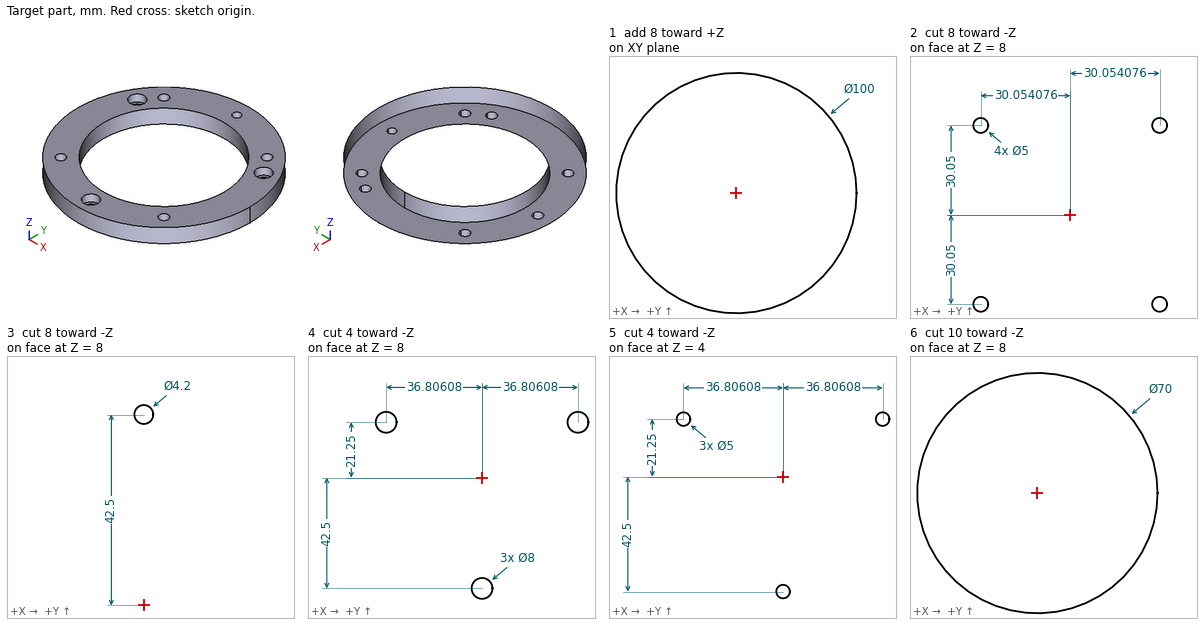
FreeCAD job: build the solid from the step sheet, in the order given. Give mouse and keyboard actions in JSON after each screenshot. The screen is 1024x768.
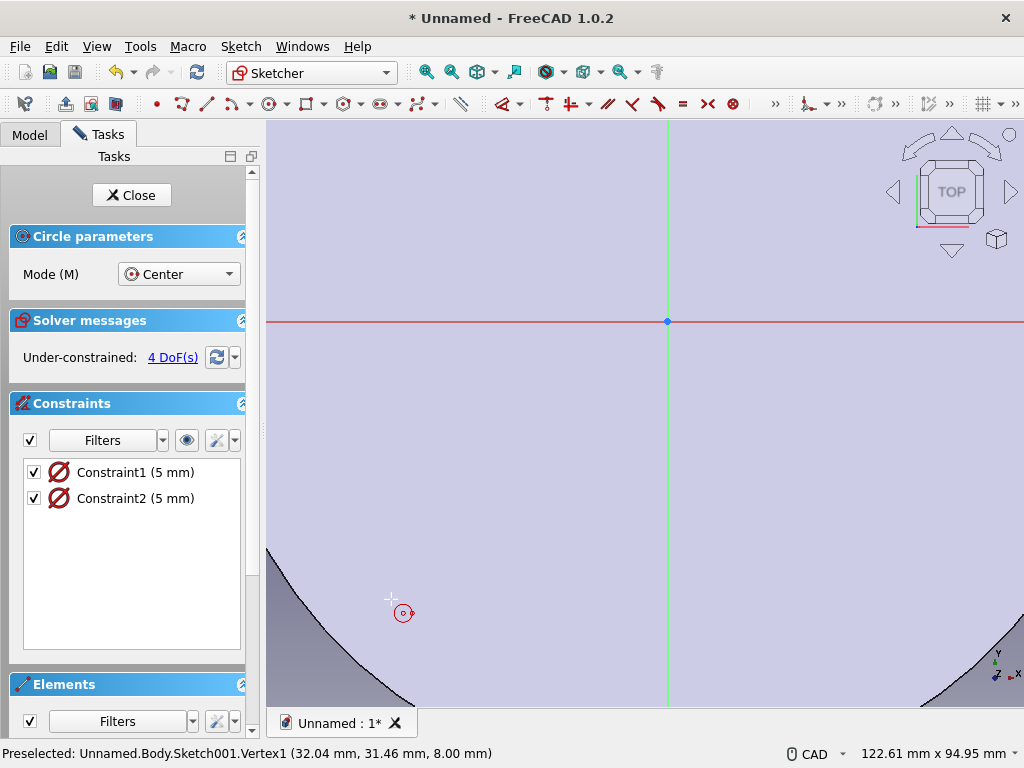
{"action": "left_click", "coordinate": [391, 599]}
{"action": "mouse_move", "coordinate": [407, 583]}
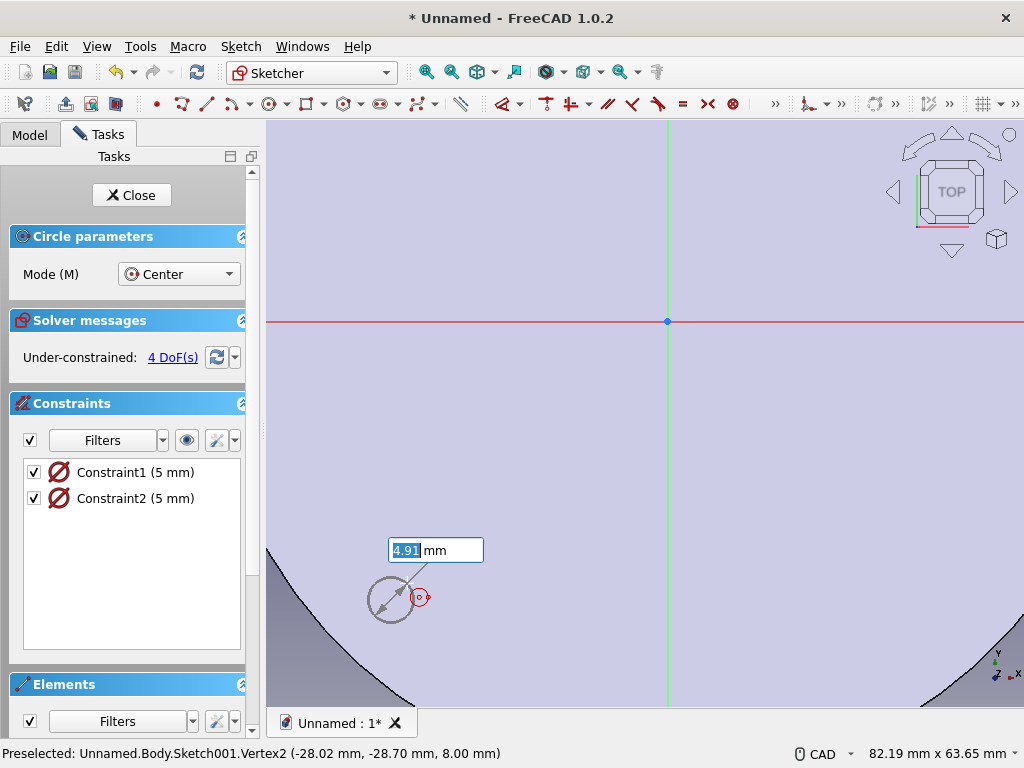
{"action": "type", "text": "5"}
{"action": "key", "text": "Return"}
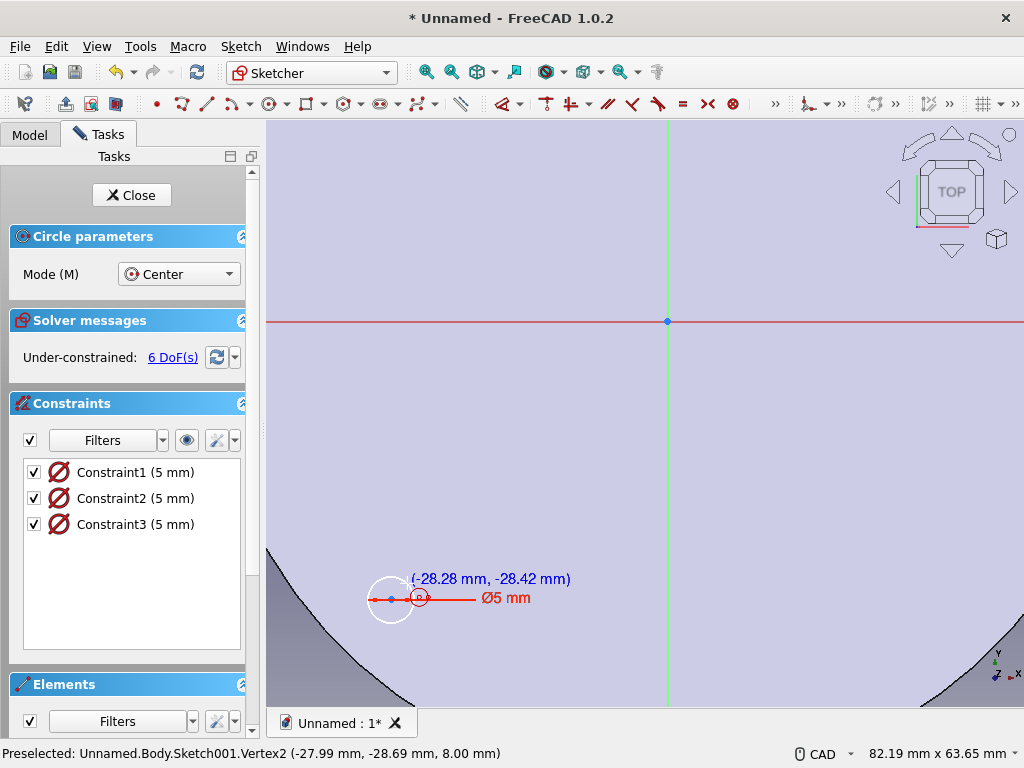
{"action": "scroll", "coordinate": [391, 600], "scroll_direction": "down", "scroll_amount": 2}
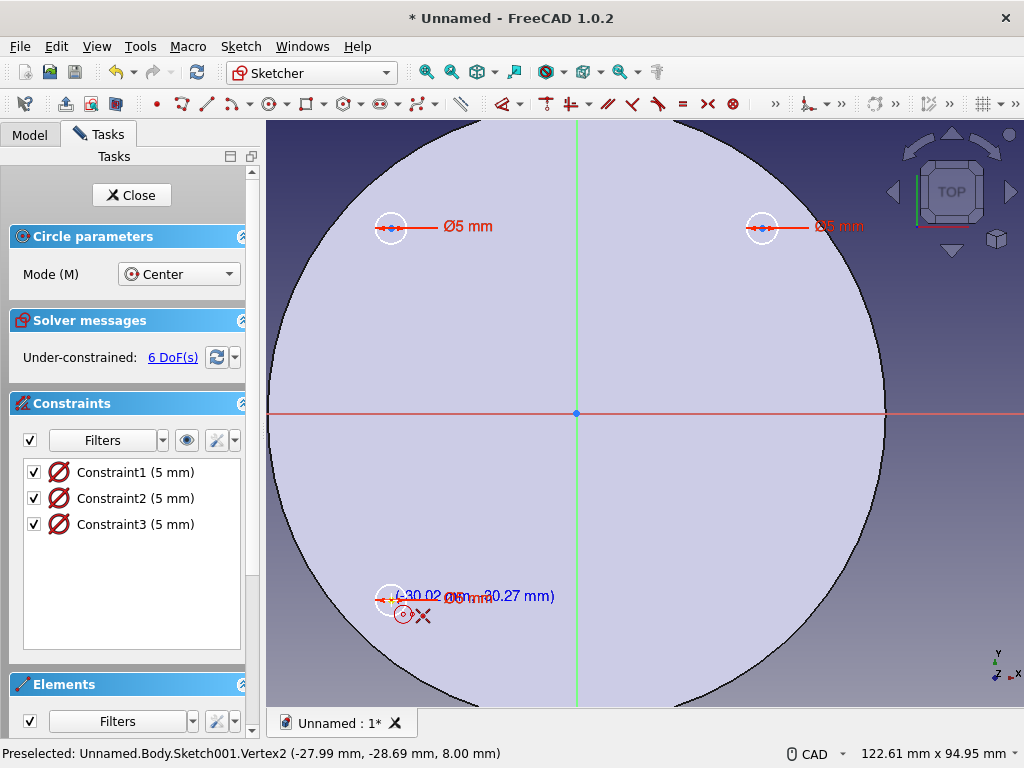
{"action": "scroll", "coordinate": [762, 600], "scroll_direction": "up", "scroll_amount": 2}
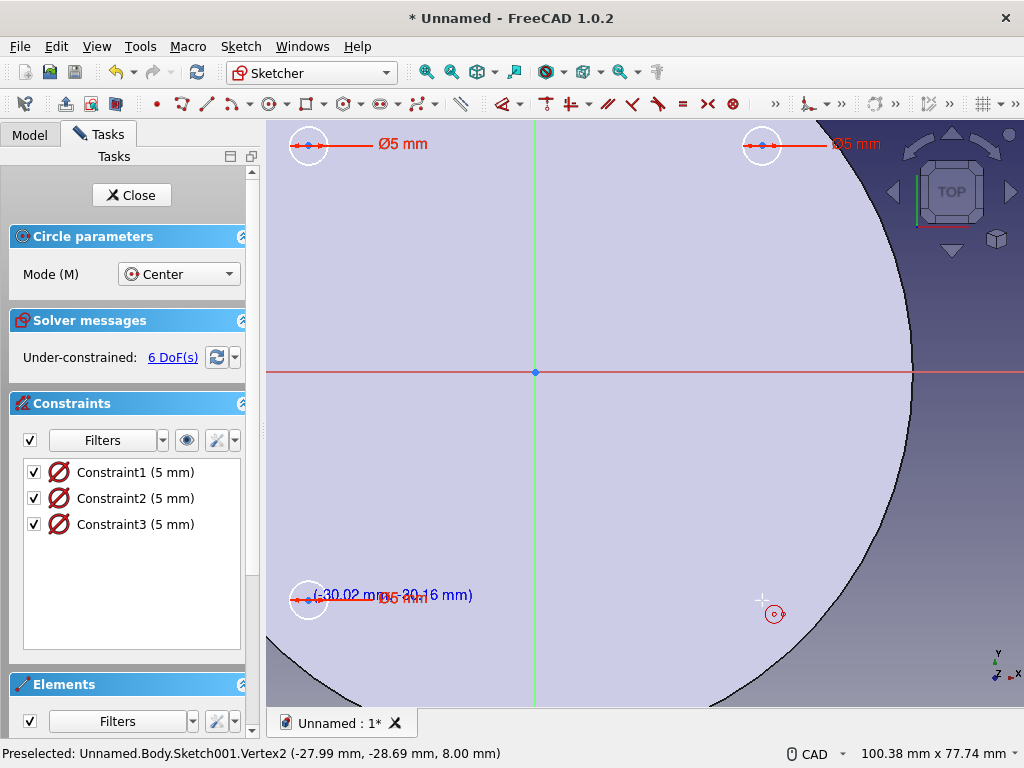
{"action": "left_click", "coordinate": [762, 599]}
{"action": "mouse_move", "coordinate": [779, 583]}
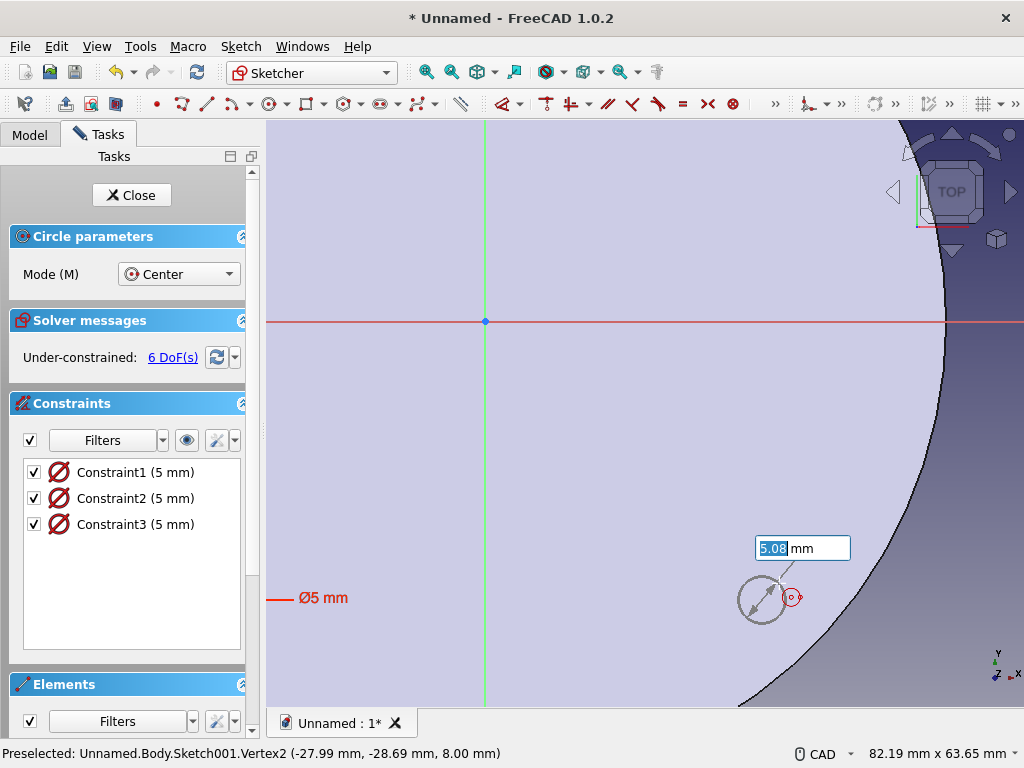
{"action": "type", "text": "5"}
{"action": "key", "text": "Return"}
{"action": "key", "text": "Escape"}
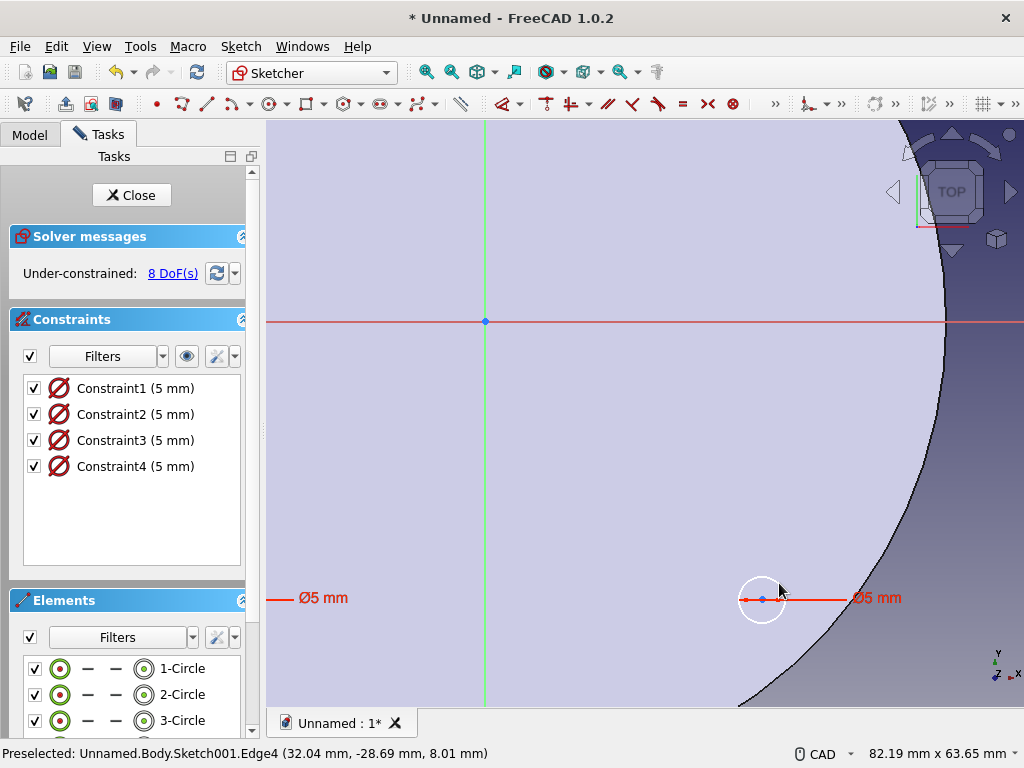
{"action": "scroll", "coordinate": [762, 600], "scroll_direction": "down", "scroll_amount": 2}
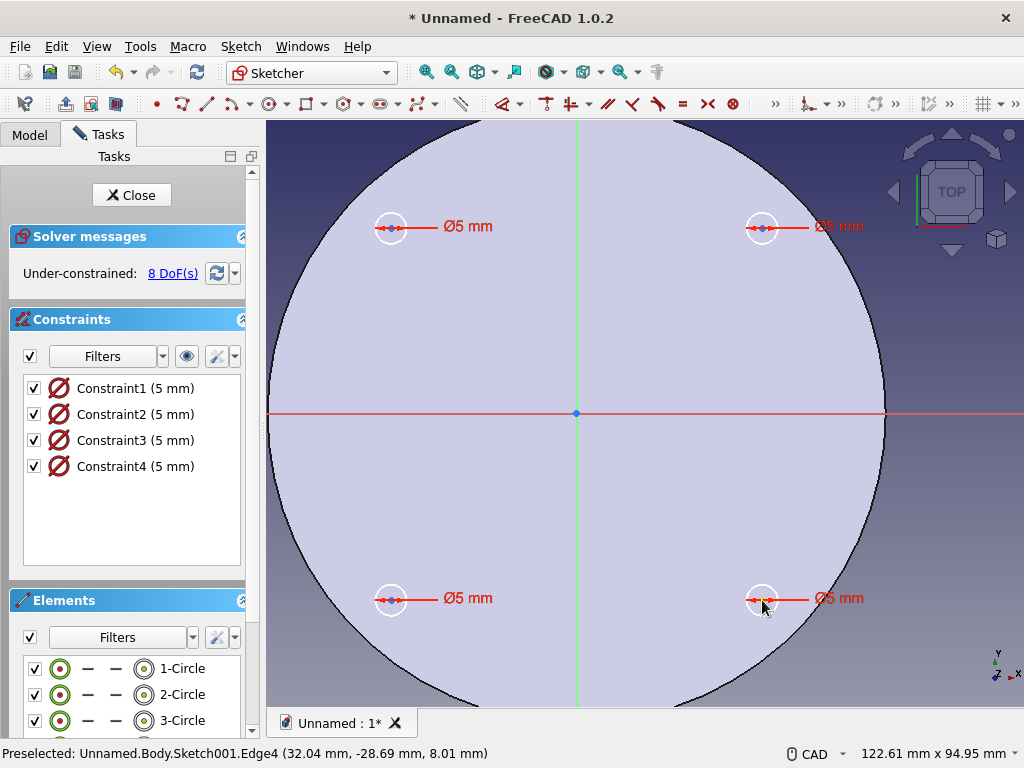
{"action": "left_click", "coordinate": [391, 228]}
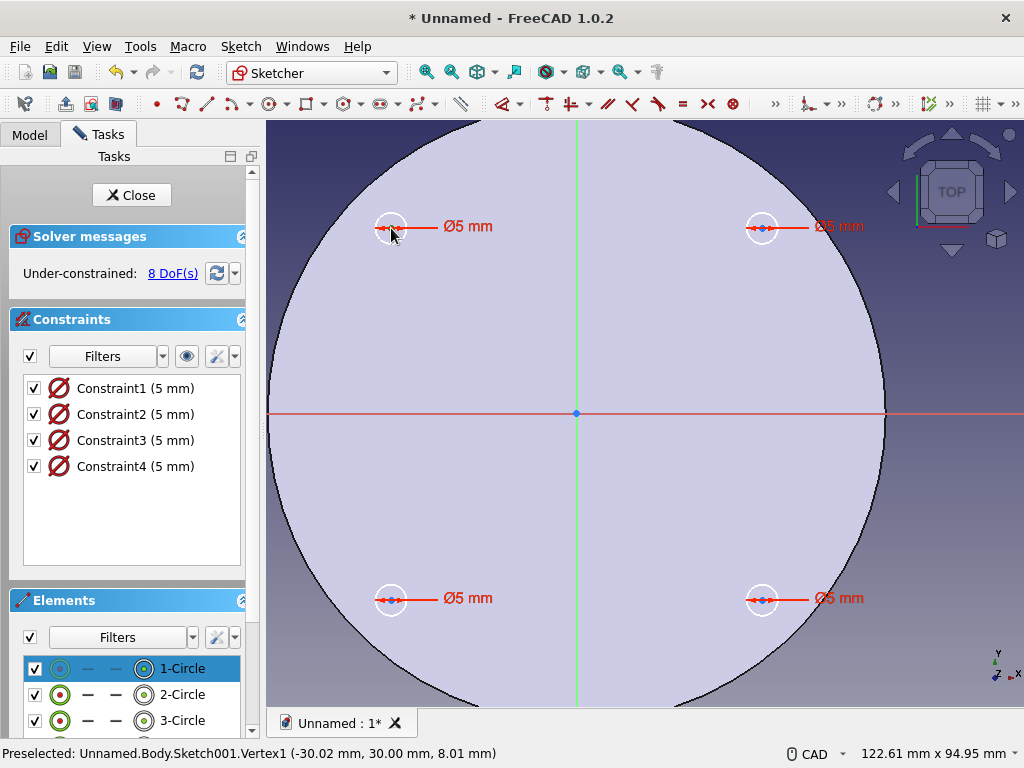
{"action": "left_click", "coordinate": [762, 228]}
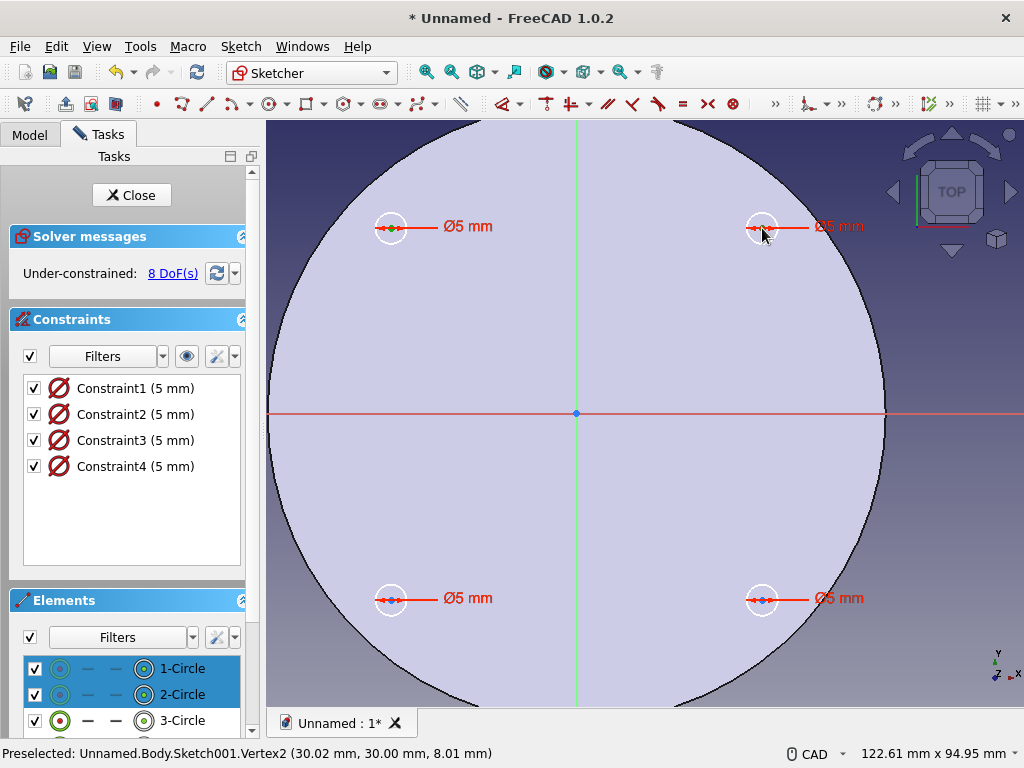
{"action": "left_click", "coordinate": [588, 104]}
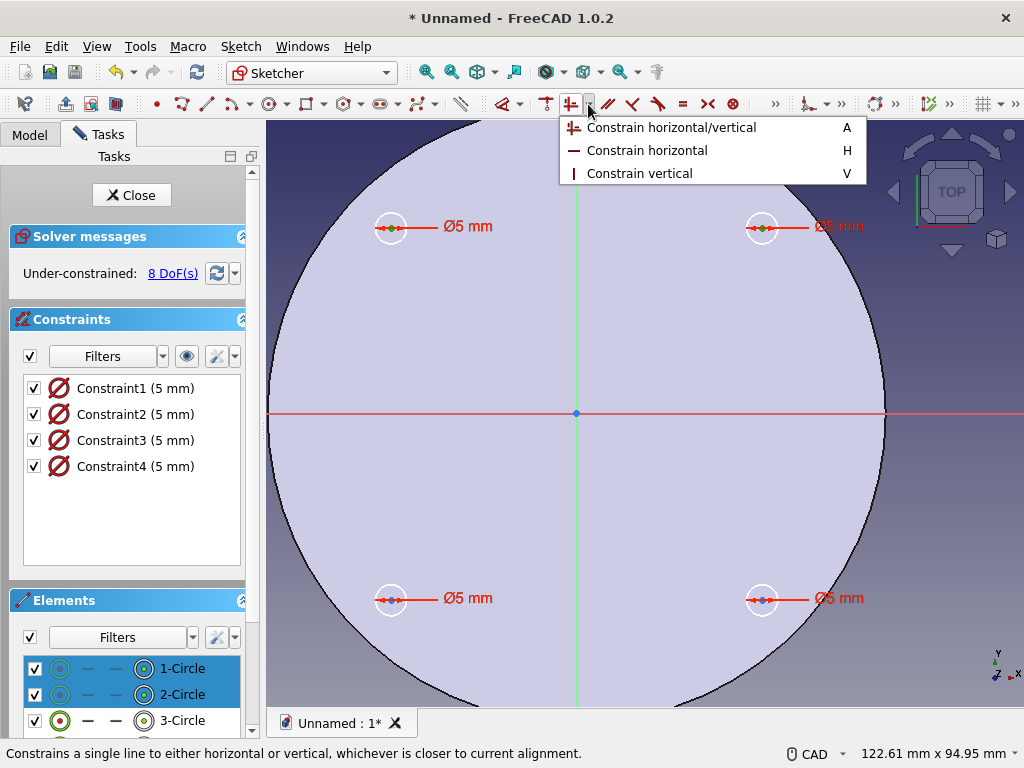
{"action": "left_click", "coordinate": [713, 150]}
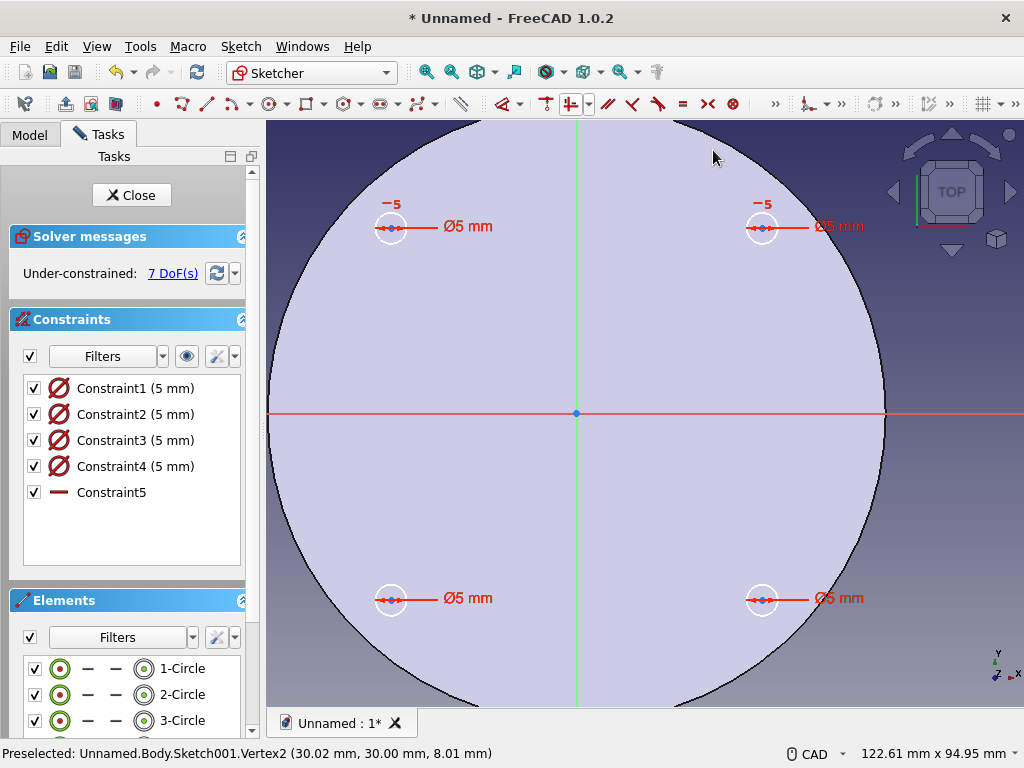
{"action": "left_click", "coordinate": [391, 228]}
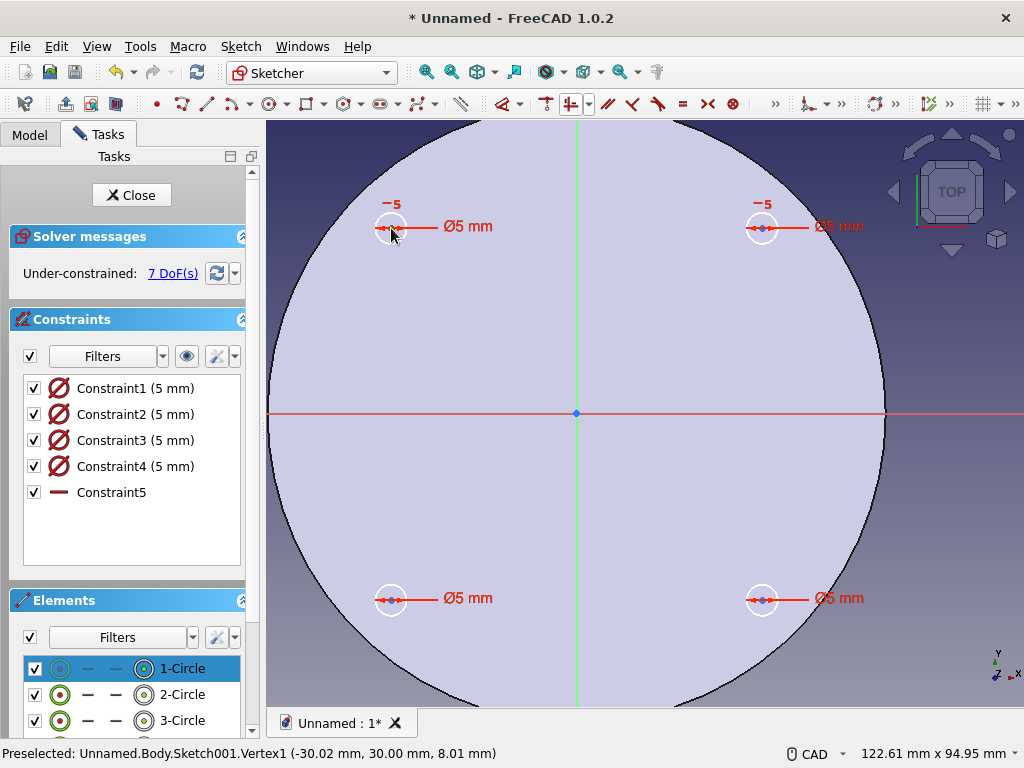
{"action": "left_click", "coordinate": [391, 600]}